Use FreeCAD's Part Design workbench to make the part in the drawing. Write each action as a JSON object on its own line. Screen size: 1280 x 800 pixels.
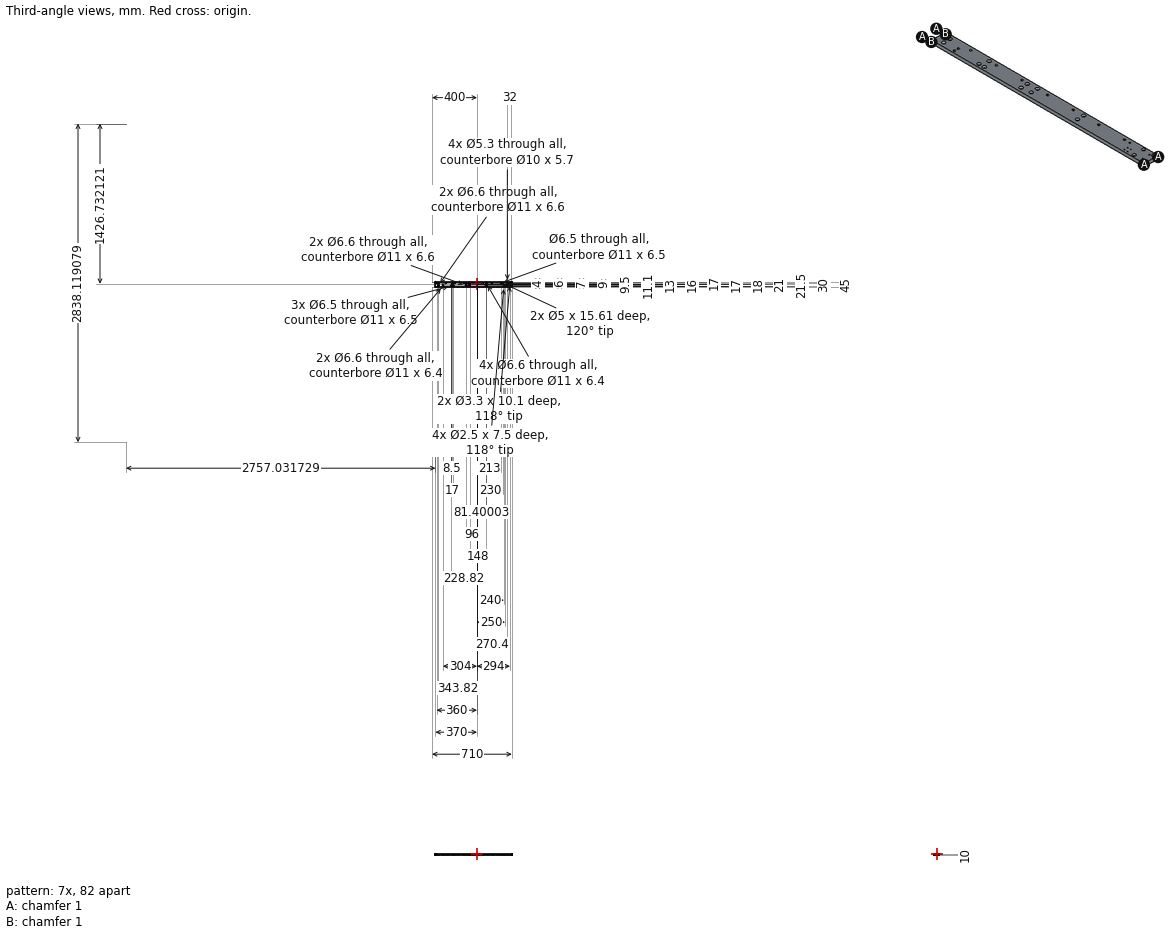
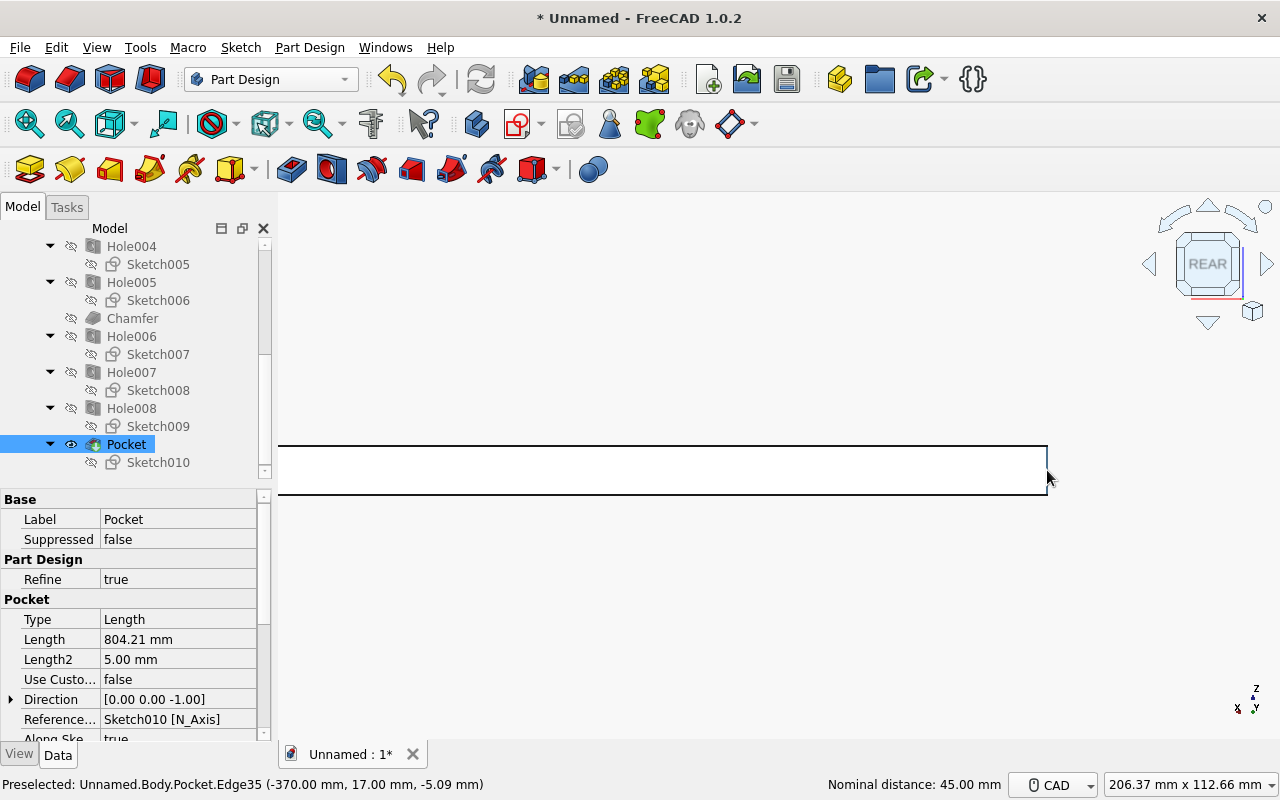
{"action": "left_click", "coordinate": [70, 80]}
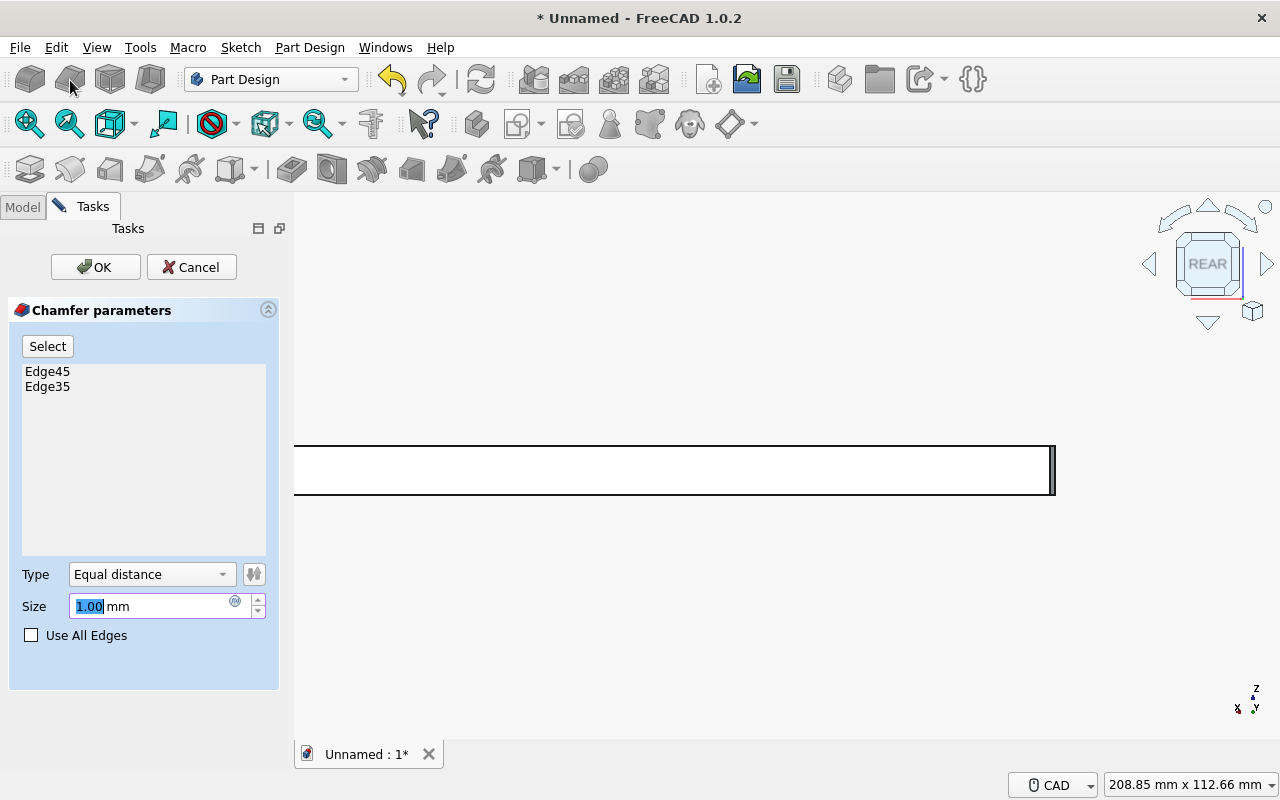
{"action": "type", "text": "1"}
{"action": "key", "text": "Tab"}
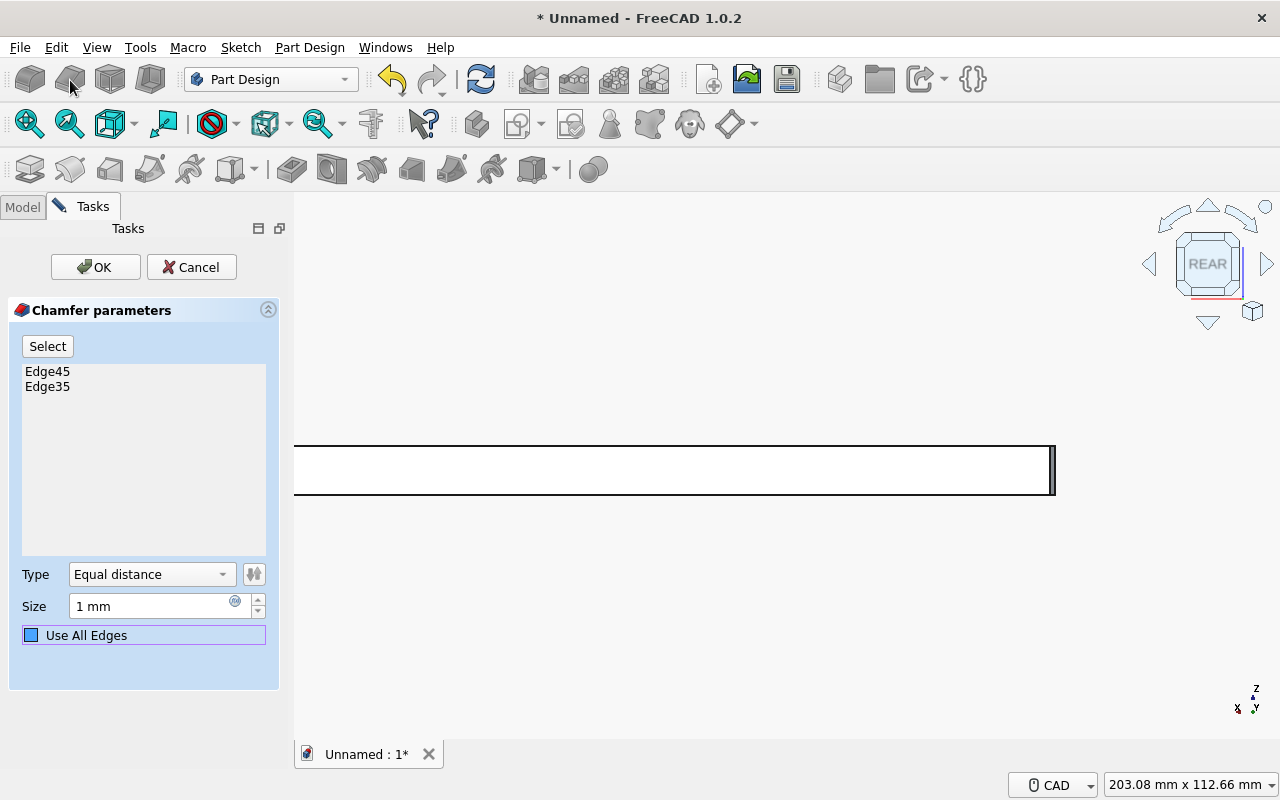
{"action": "left_click", "coordinate": [96, 267]}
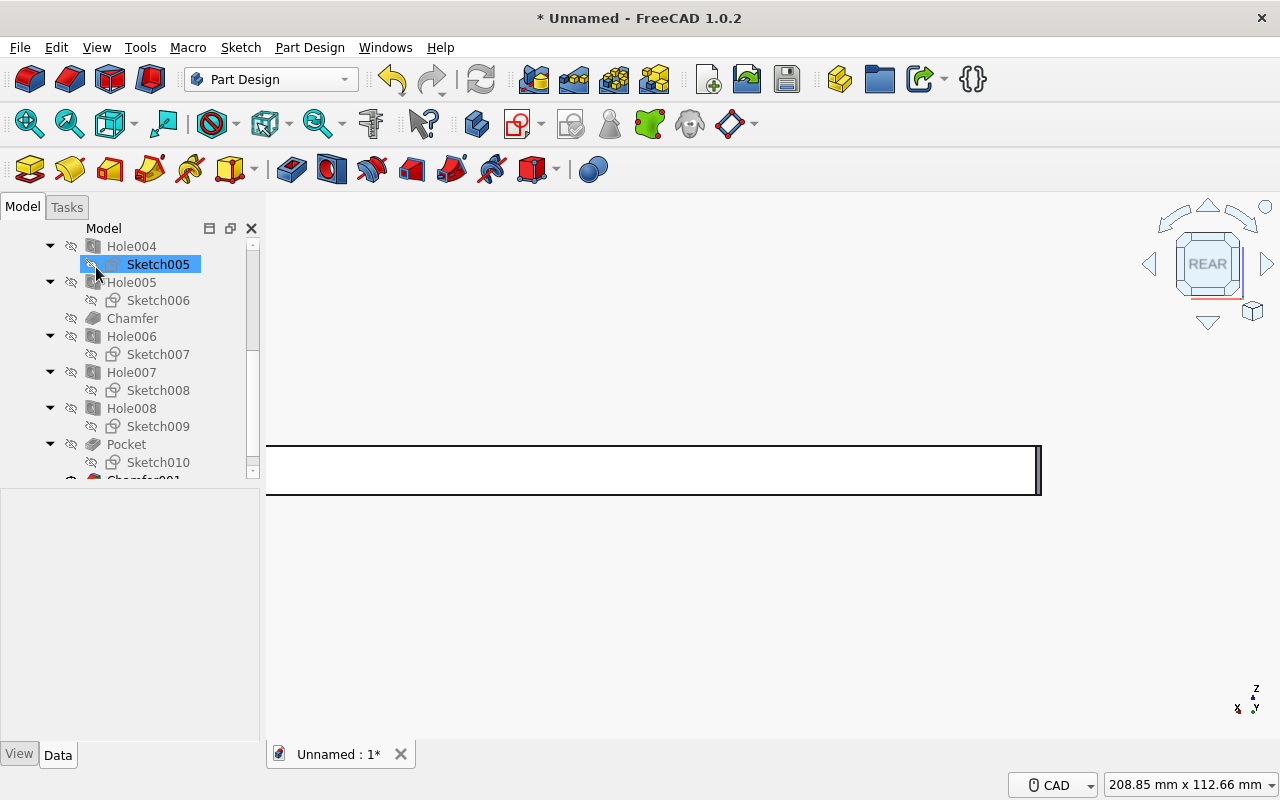
{"action": "left_click", "coordinate": [30, 124]}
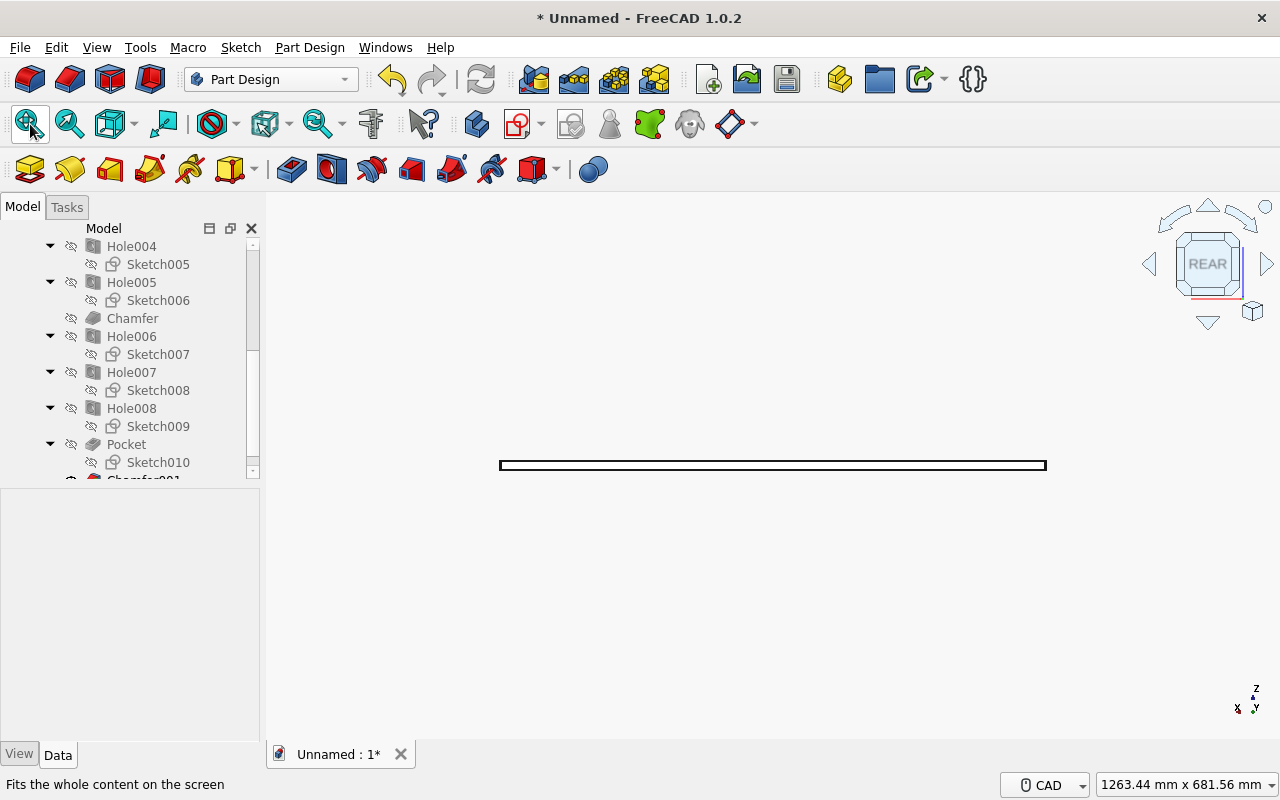
{"action": "key", "text": "0"}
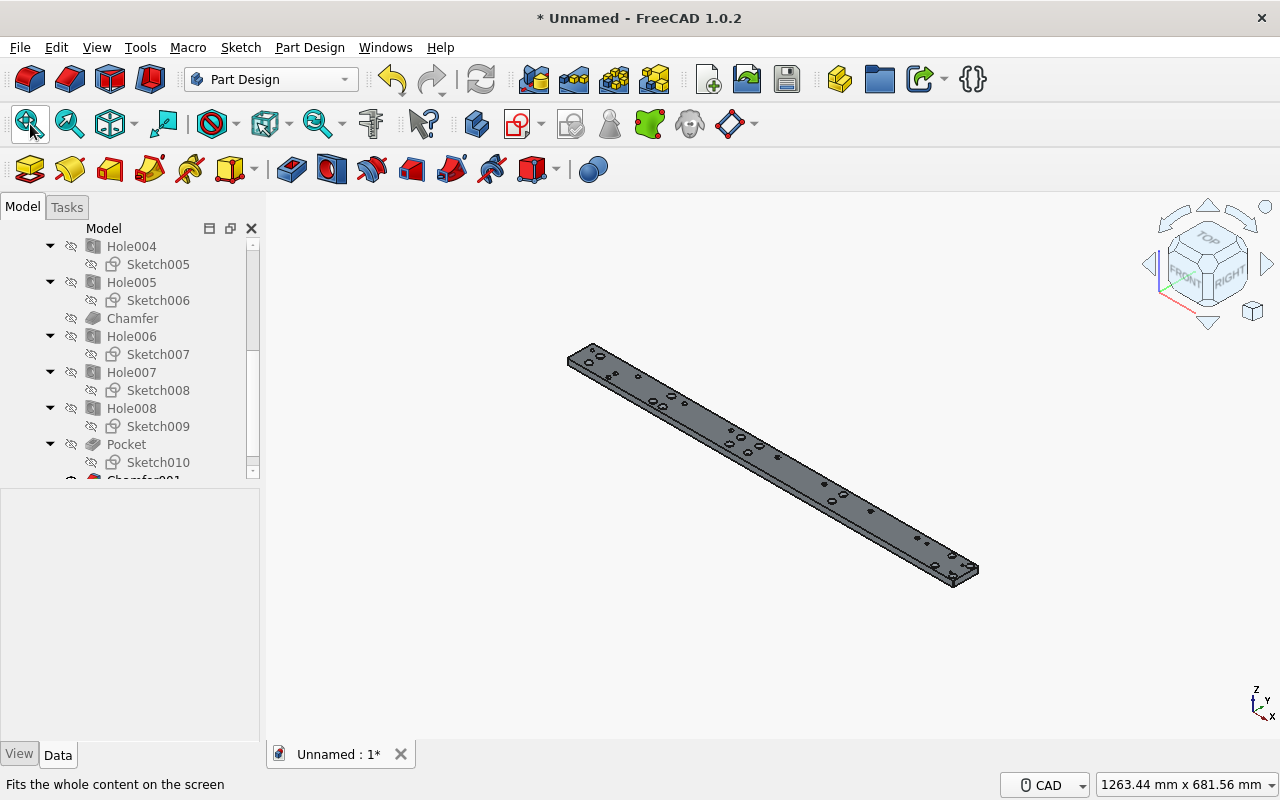
{"action": "left_click", "coordinate": [30, 124]}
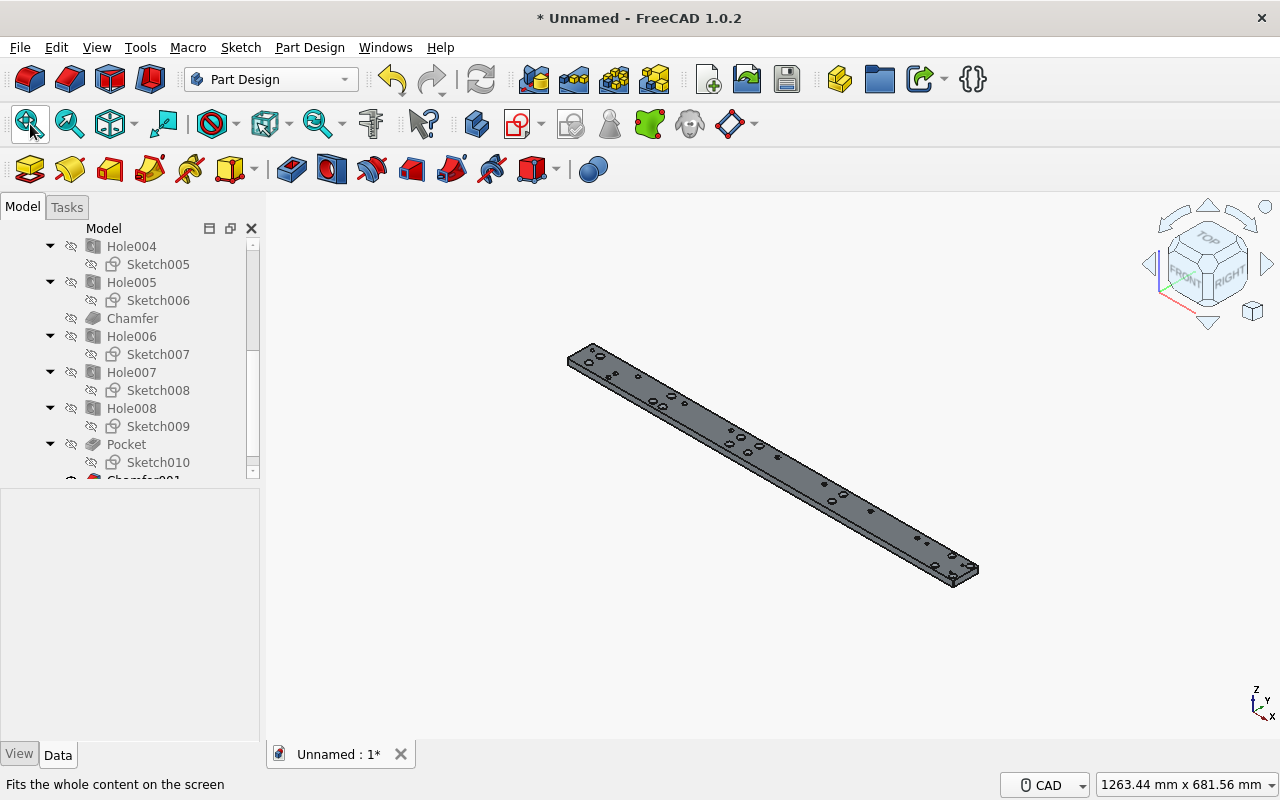
{"action": "left_click", "coordinate": [883, 525]}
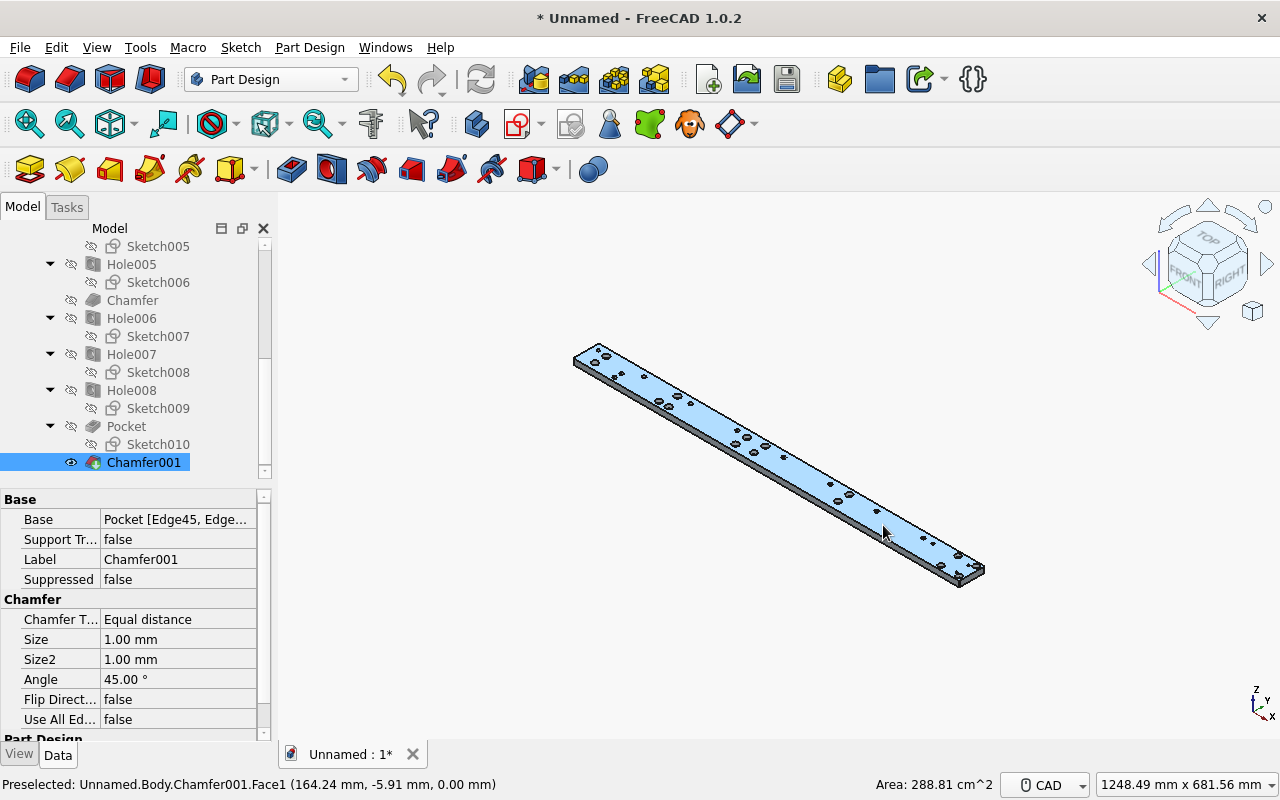
{"action": "left_click", "coordinate": [518, 124]}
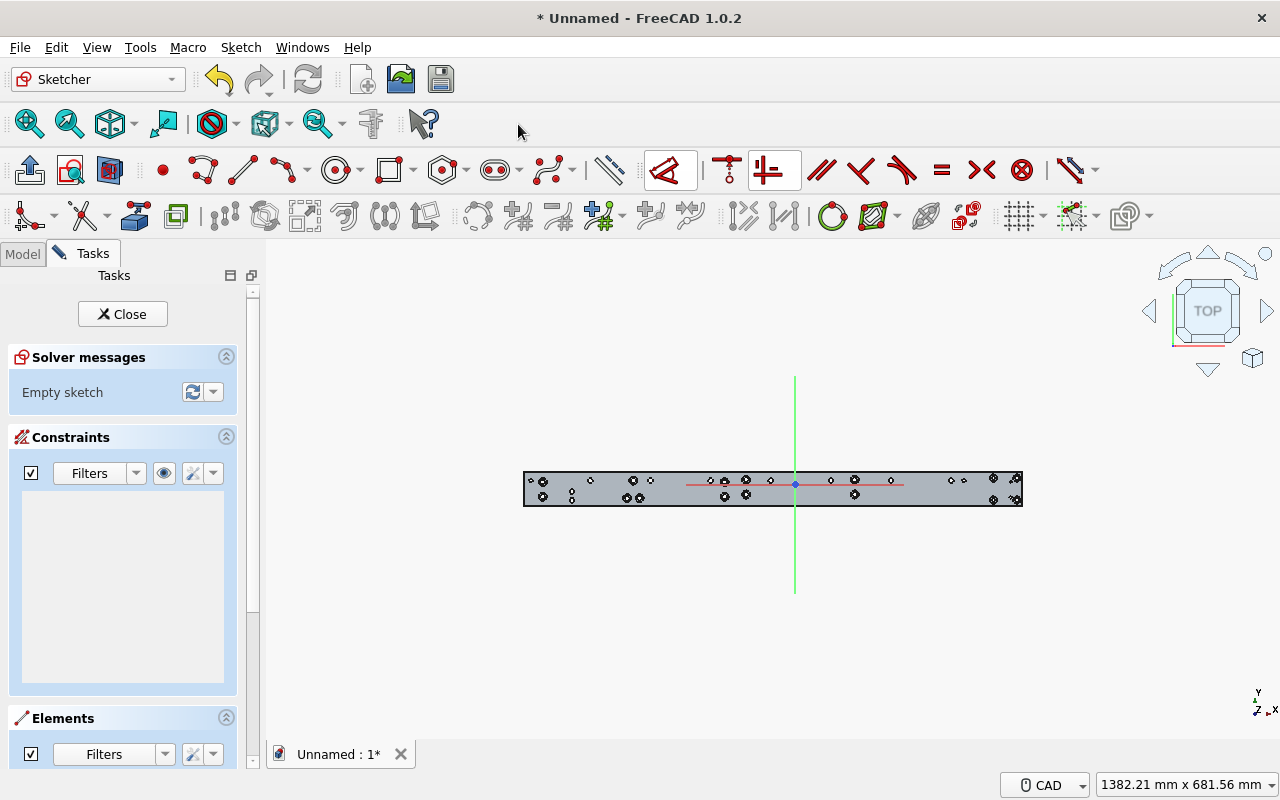
{"action": "scroll", "coordinate": [989, 497], "scroll_direction": "up", "scroll_amount": 15}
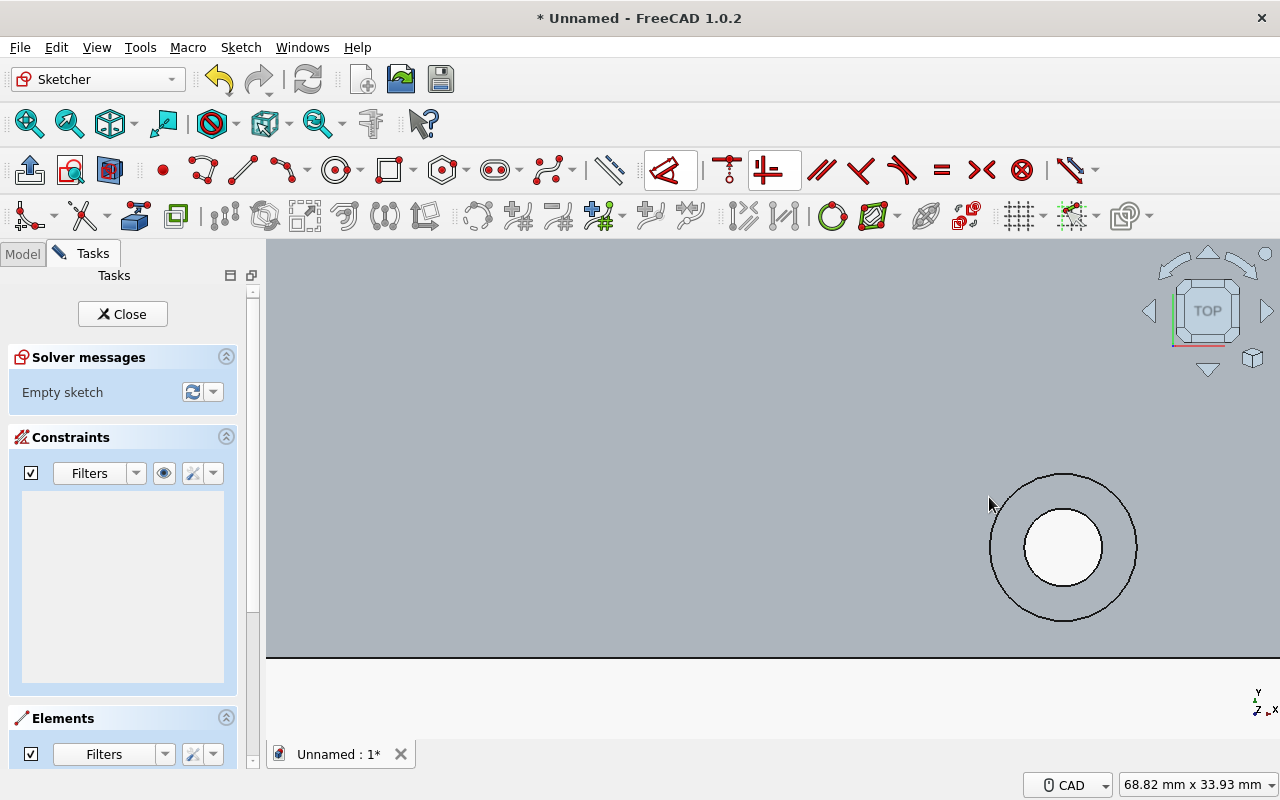
{"action": "scroll", "coordinate": [658, 479], "scroll_direction": "up", "scroll_amount": 2}